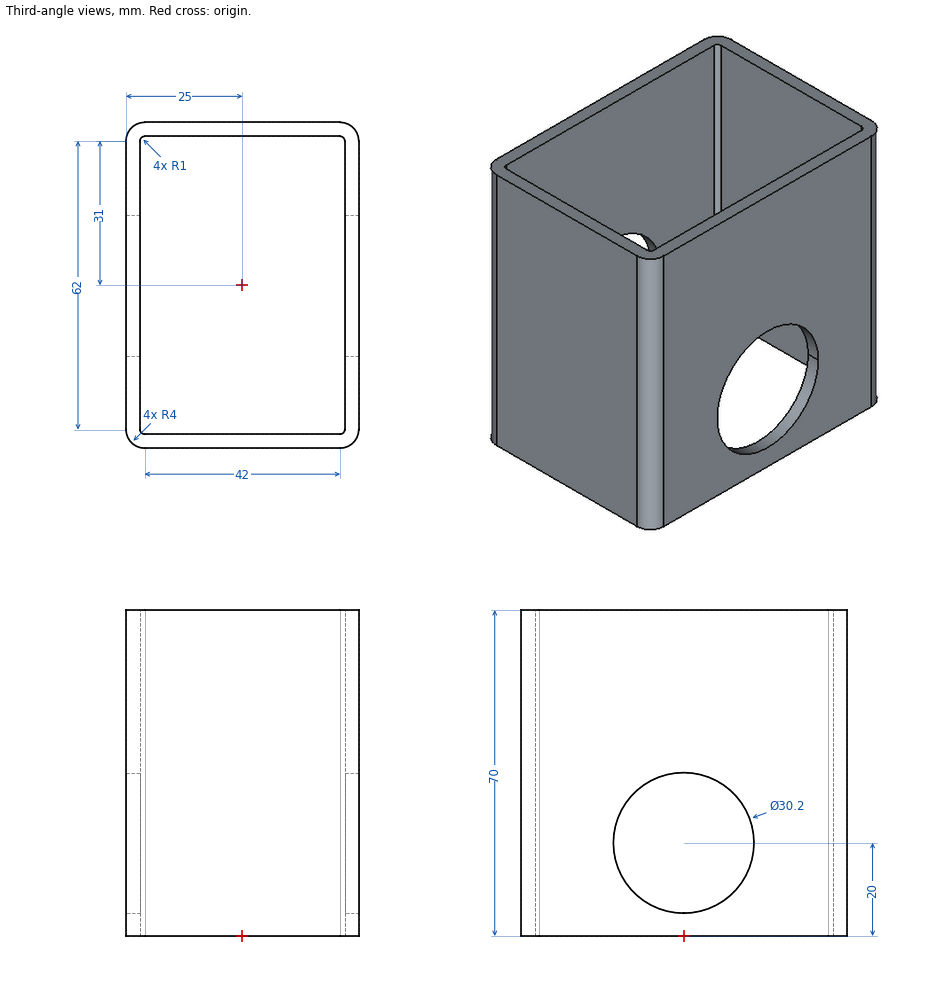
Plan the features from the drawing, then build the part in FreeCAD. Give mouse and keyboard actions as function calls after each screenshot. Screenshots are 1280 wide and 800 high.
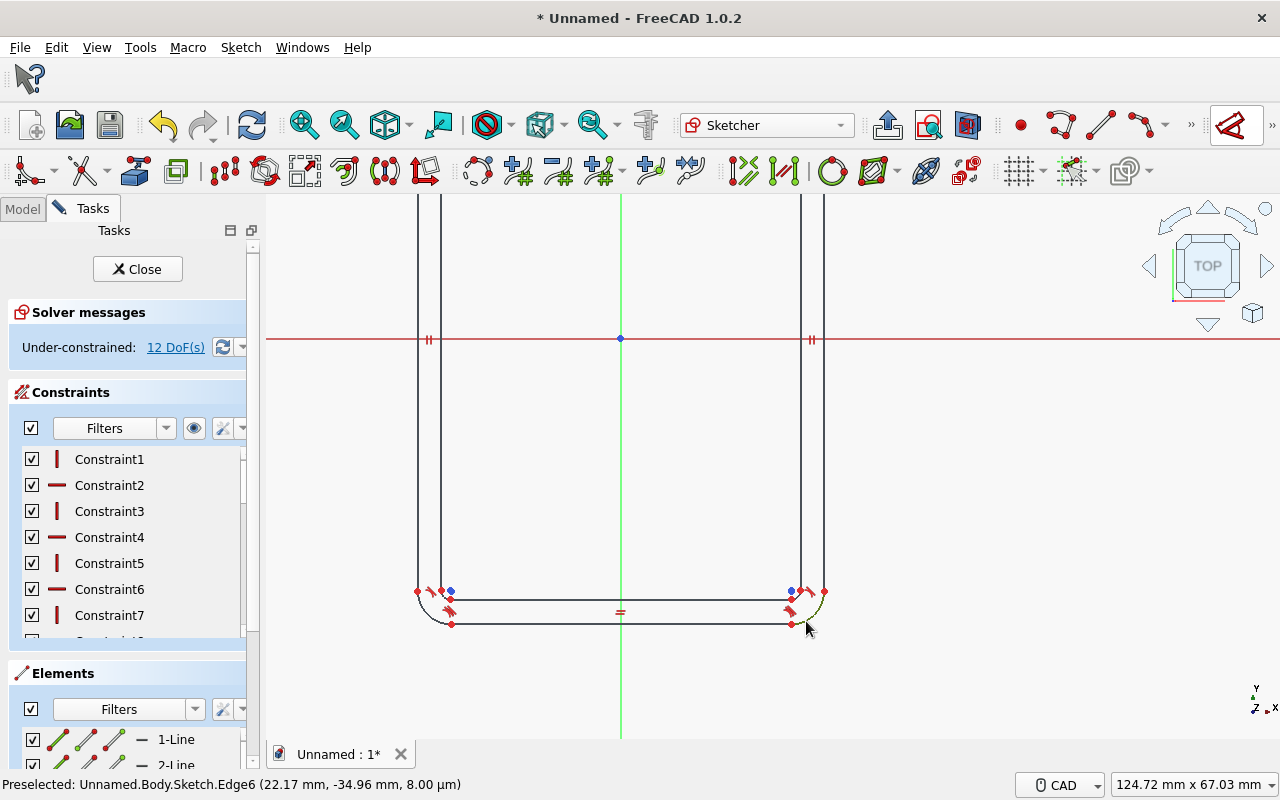
scroll(798, 597, up, 4)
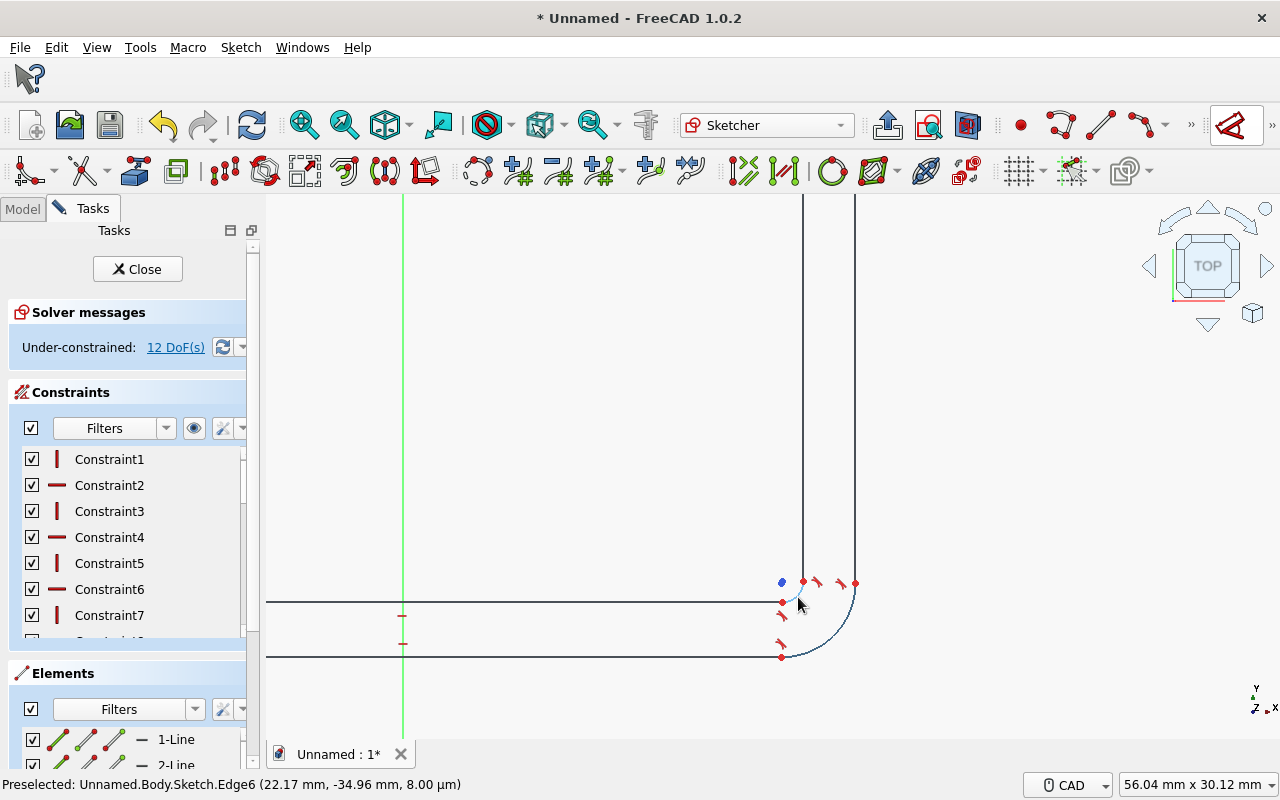
click(797, 596)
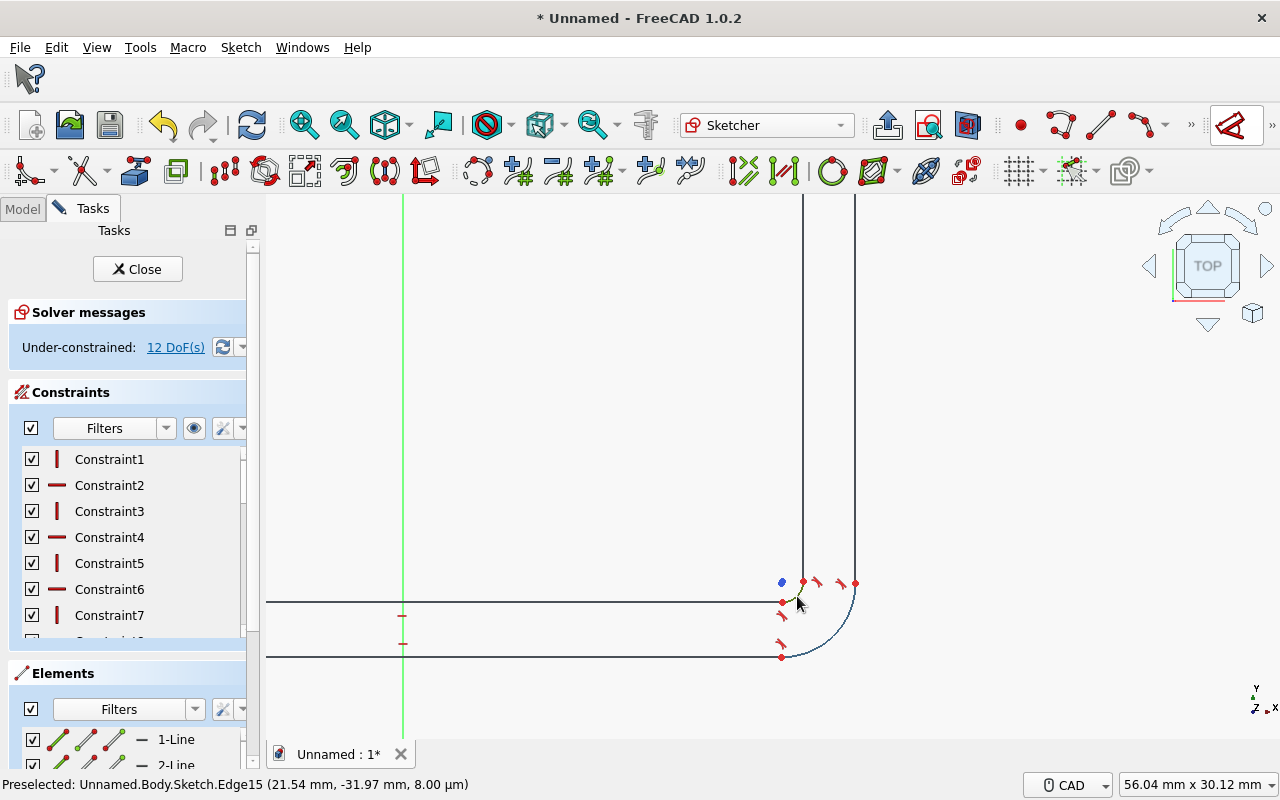
key(c)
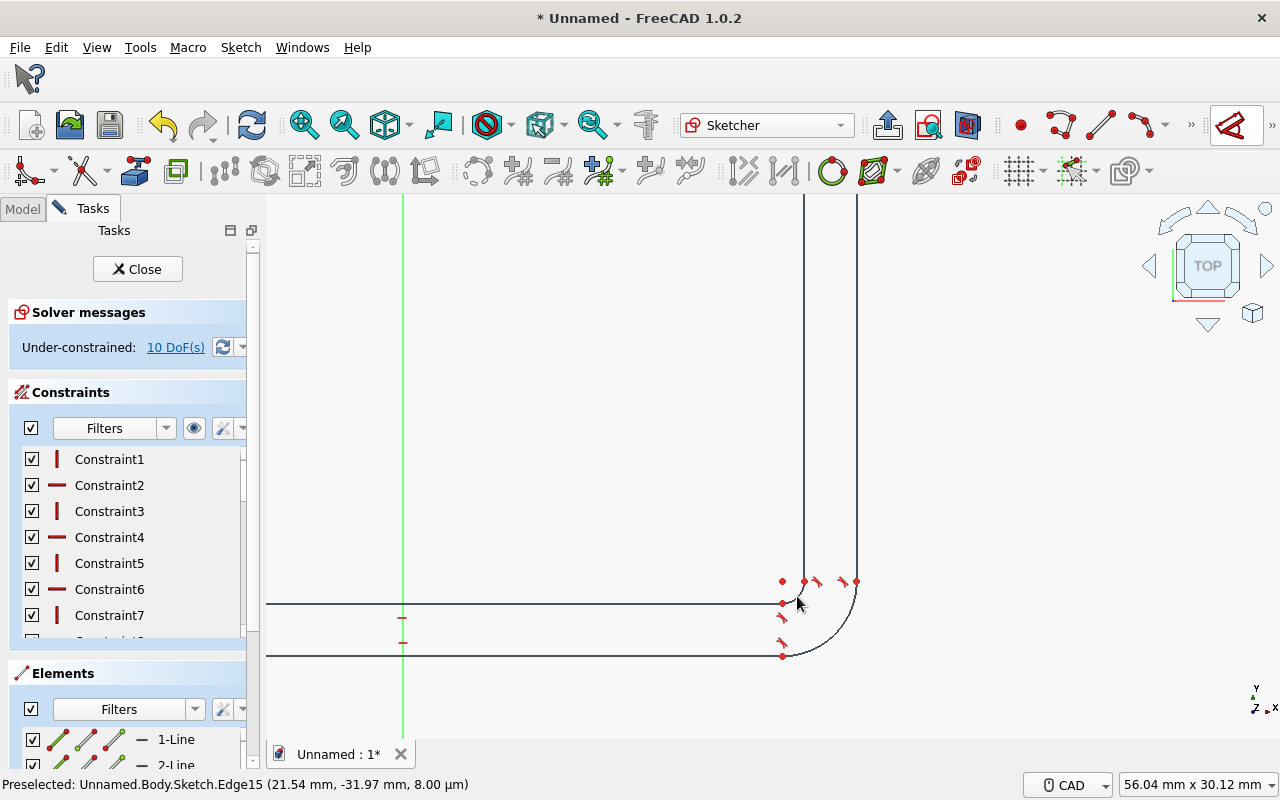
scroll(803, 612, down, 7)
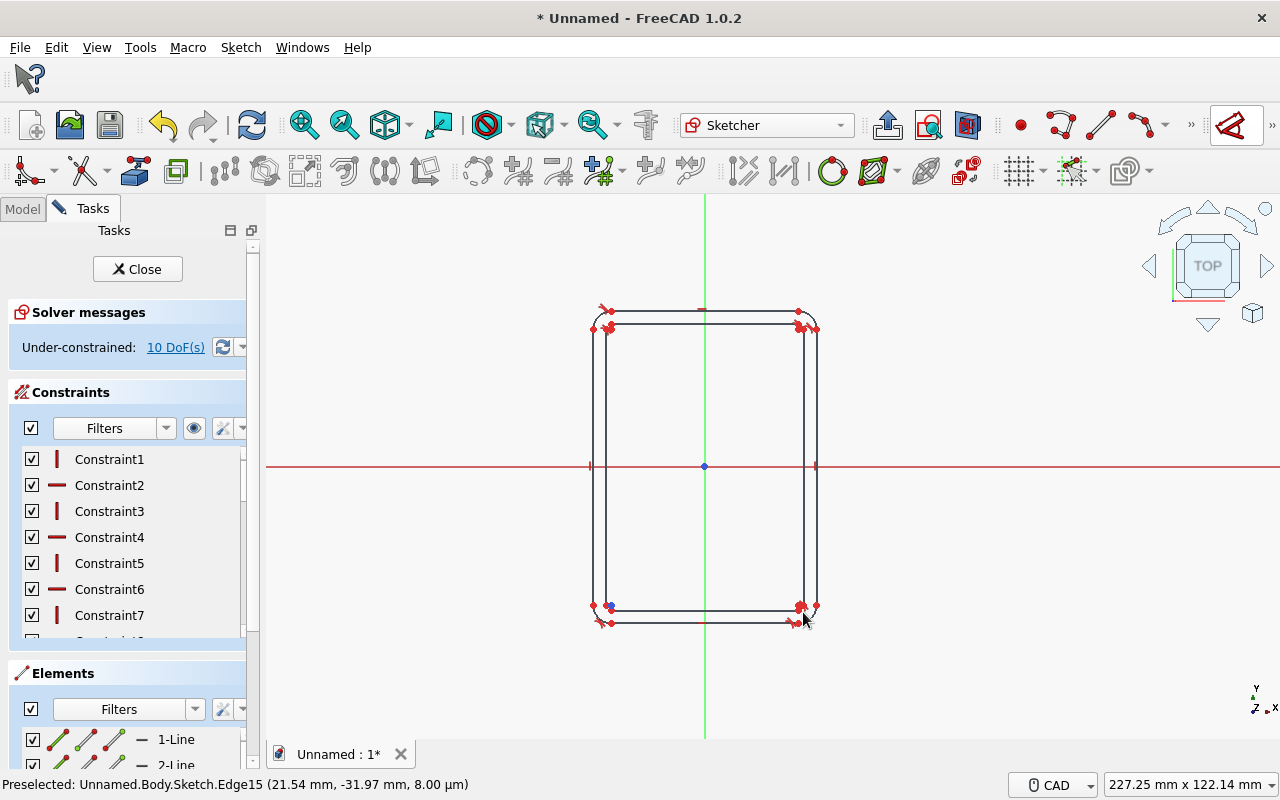
scroll(595, 613, up, 3)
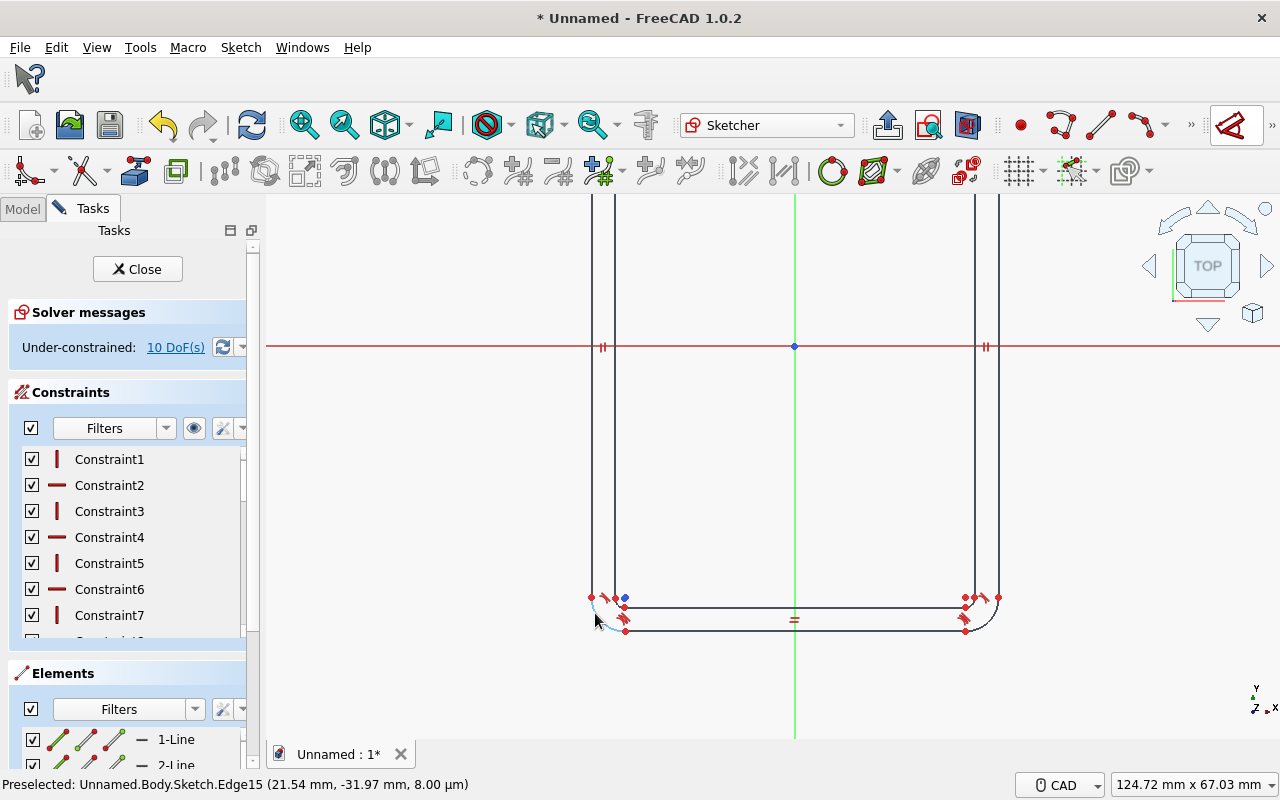
click(595, 613)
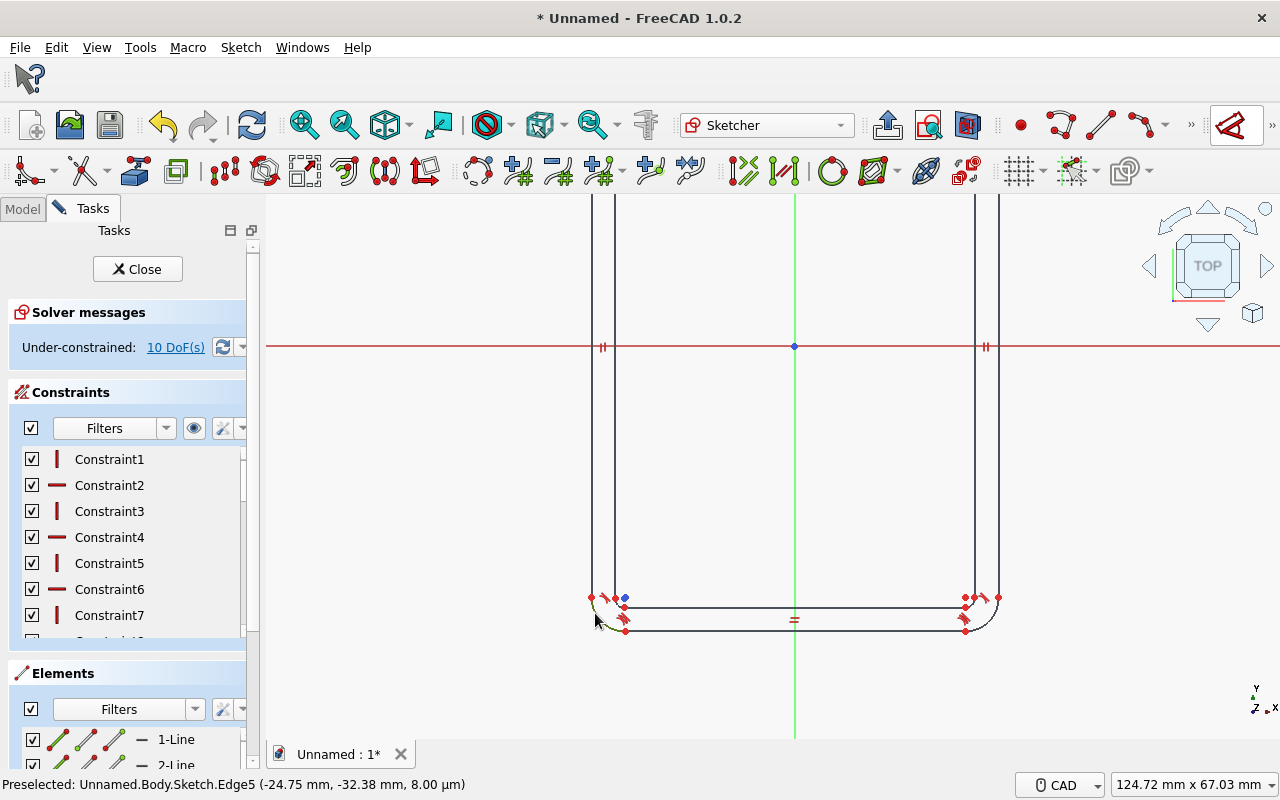
click(980, 628)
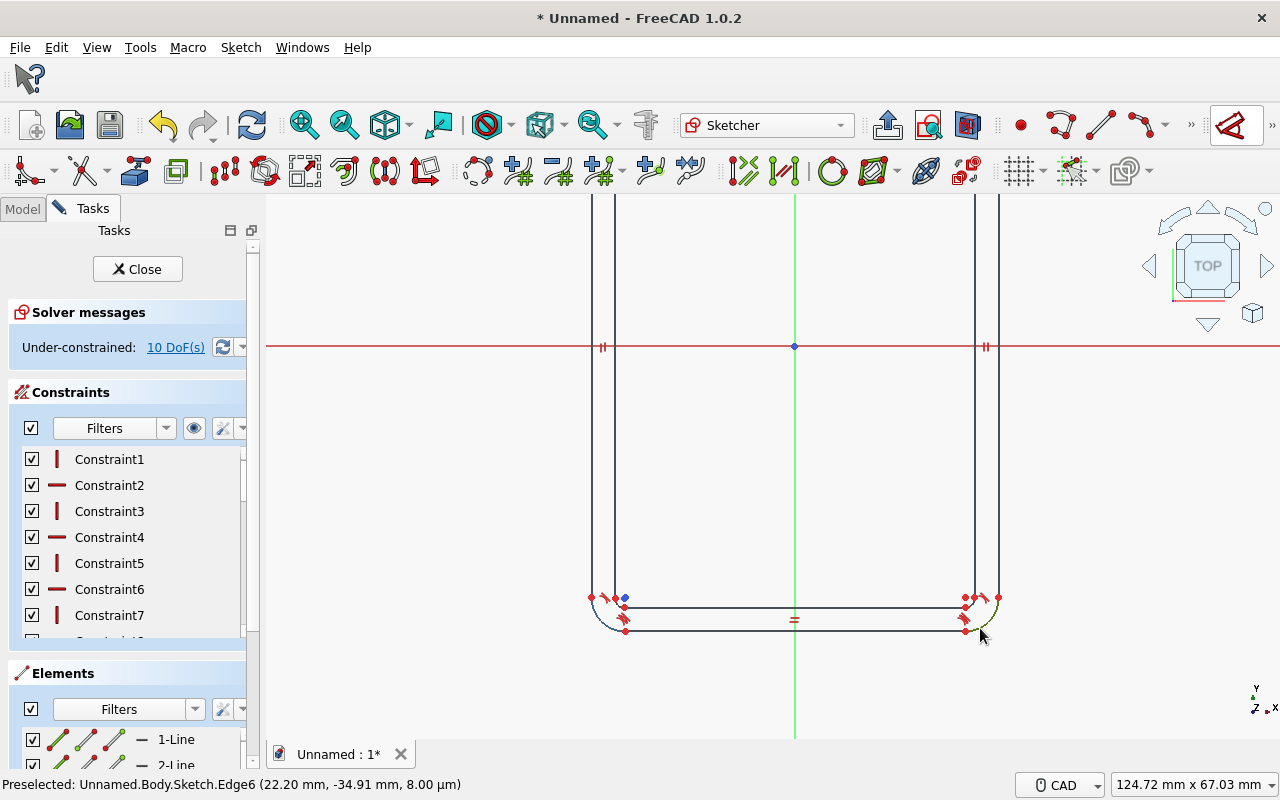
scroll(595, 613, down, 3)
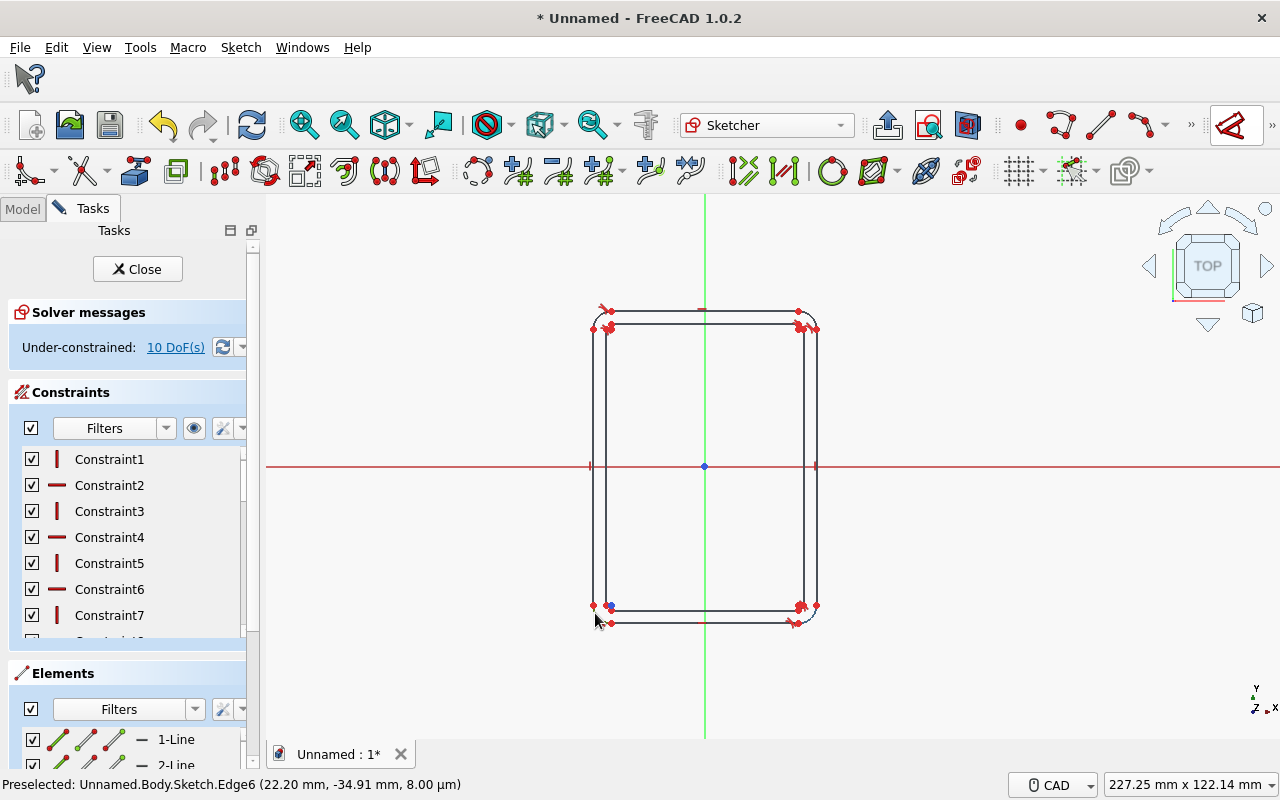
scroll(815, 321, up, 3)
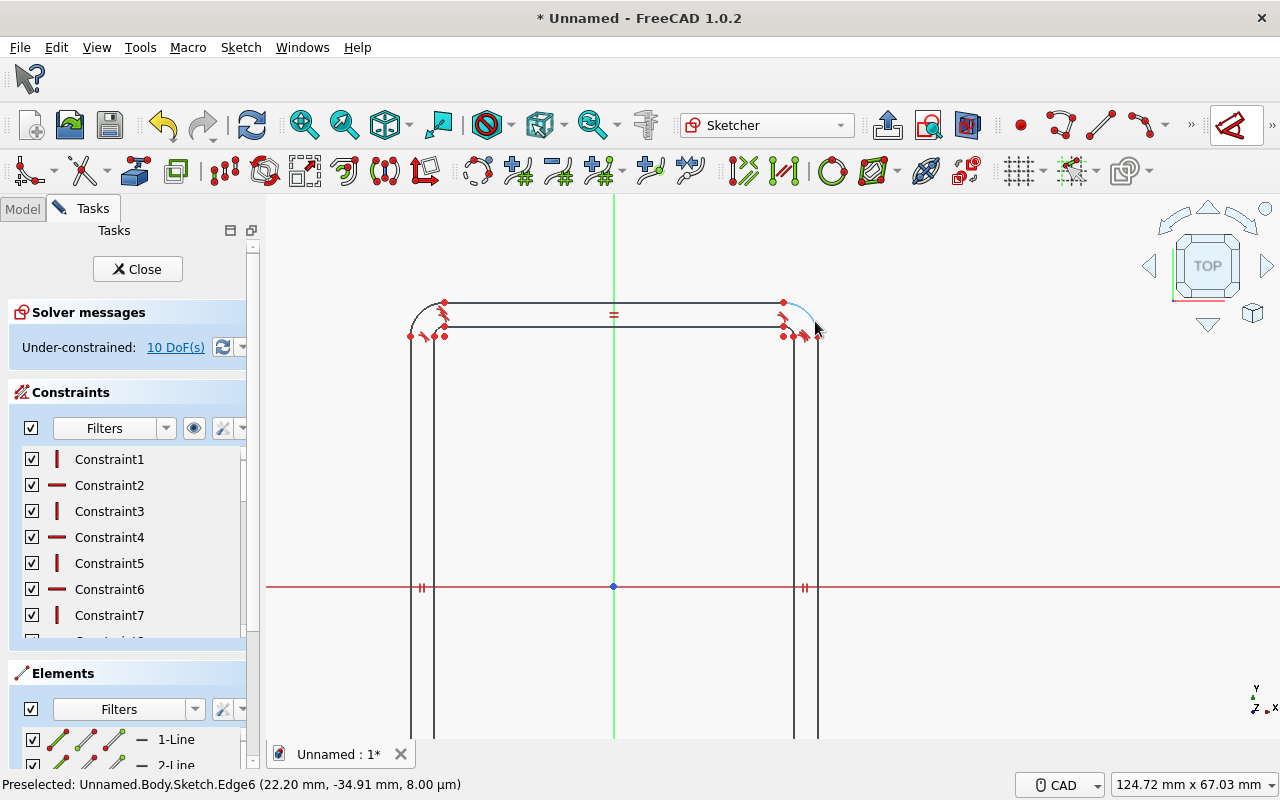
click(814, 321)